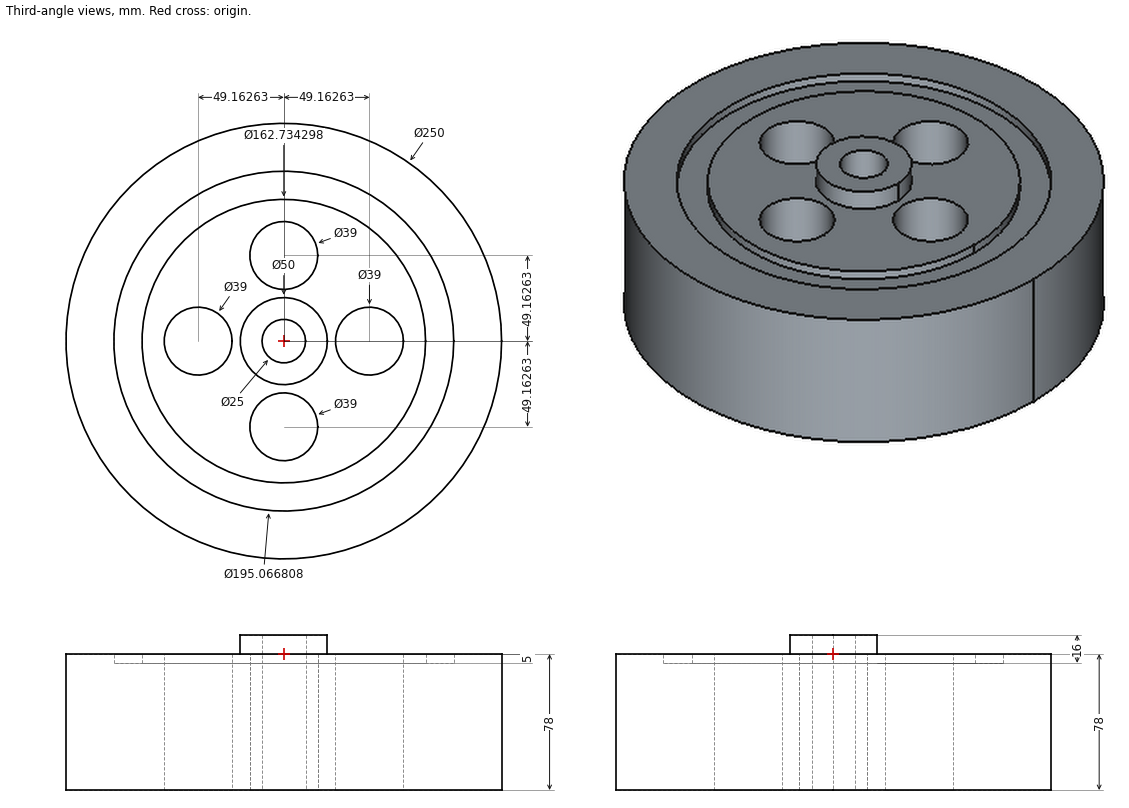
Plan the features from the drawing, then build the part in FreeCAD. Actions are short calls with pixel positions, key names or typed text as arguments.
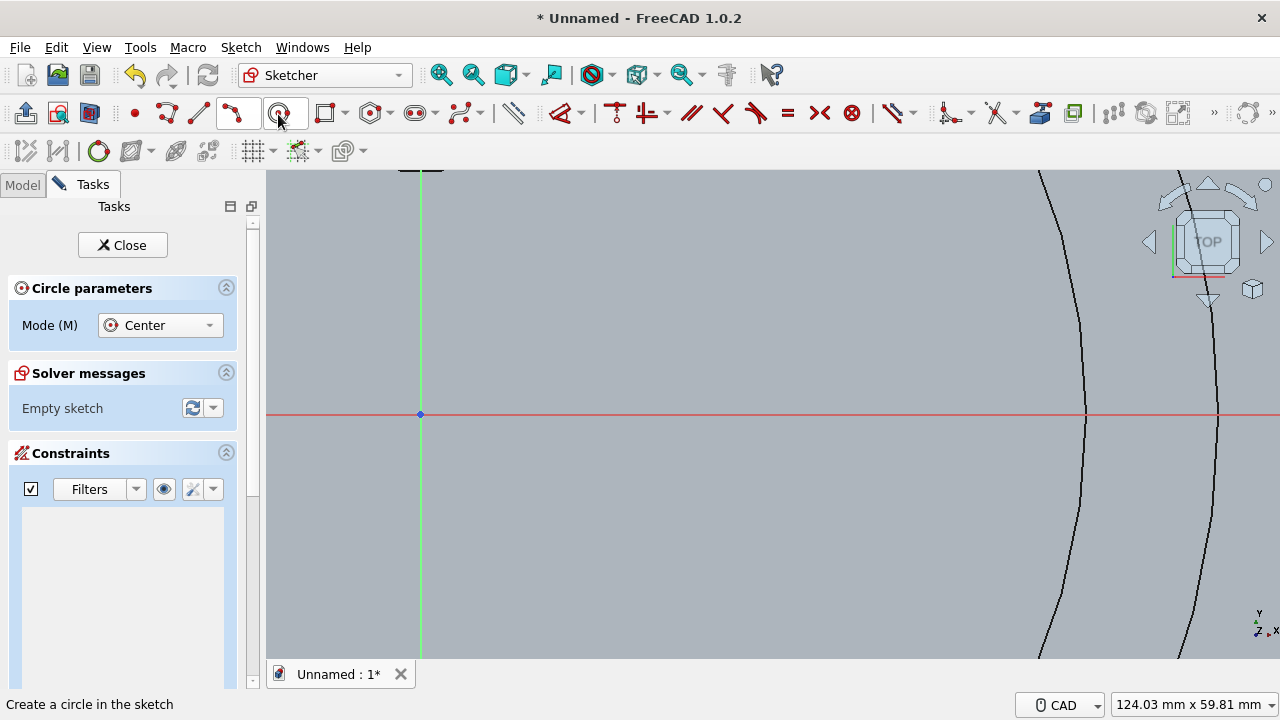
click(823, 414)
move(936, 302)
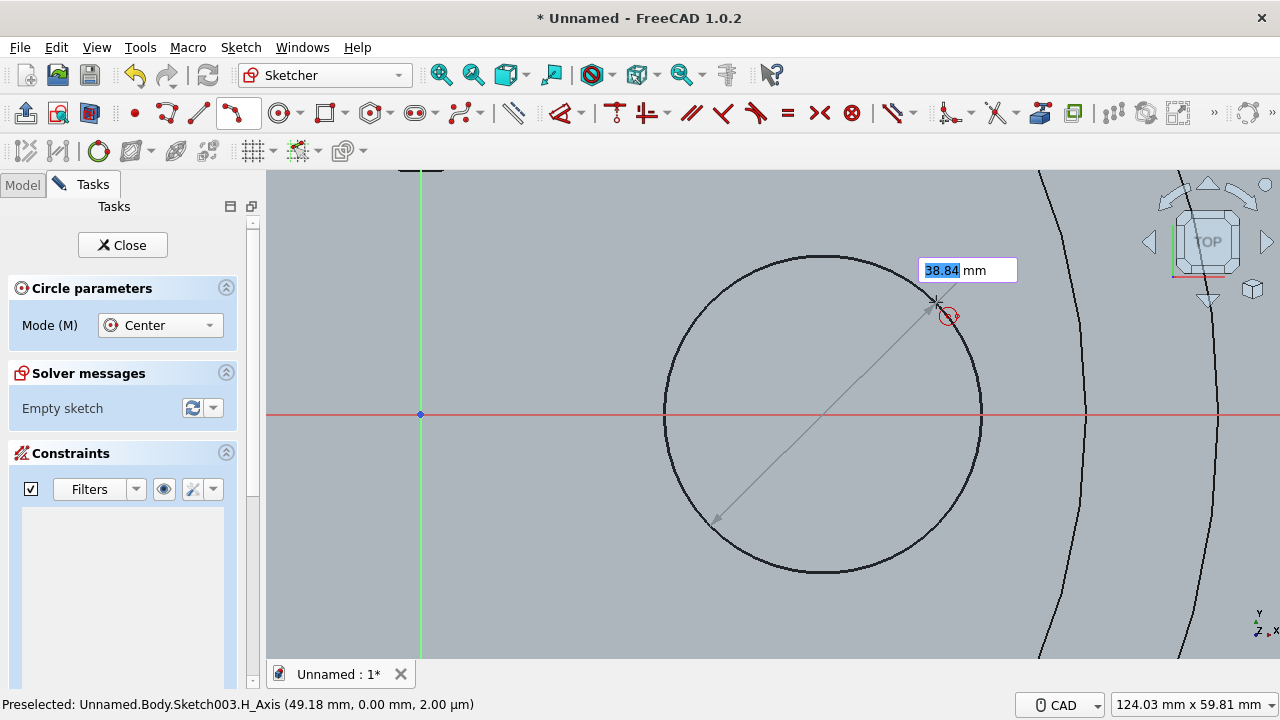
text(39)
key(Return)
key(Escape)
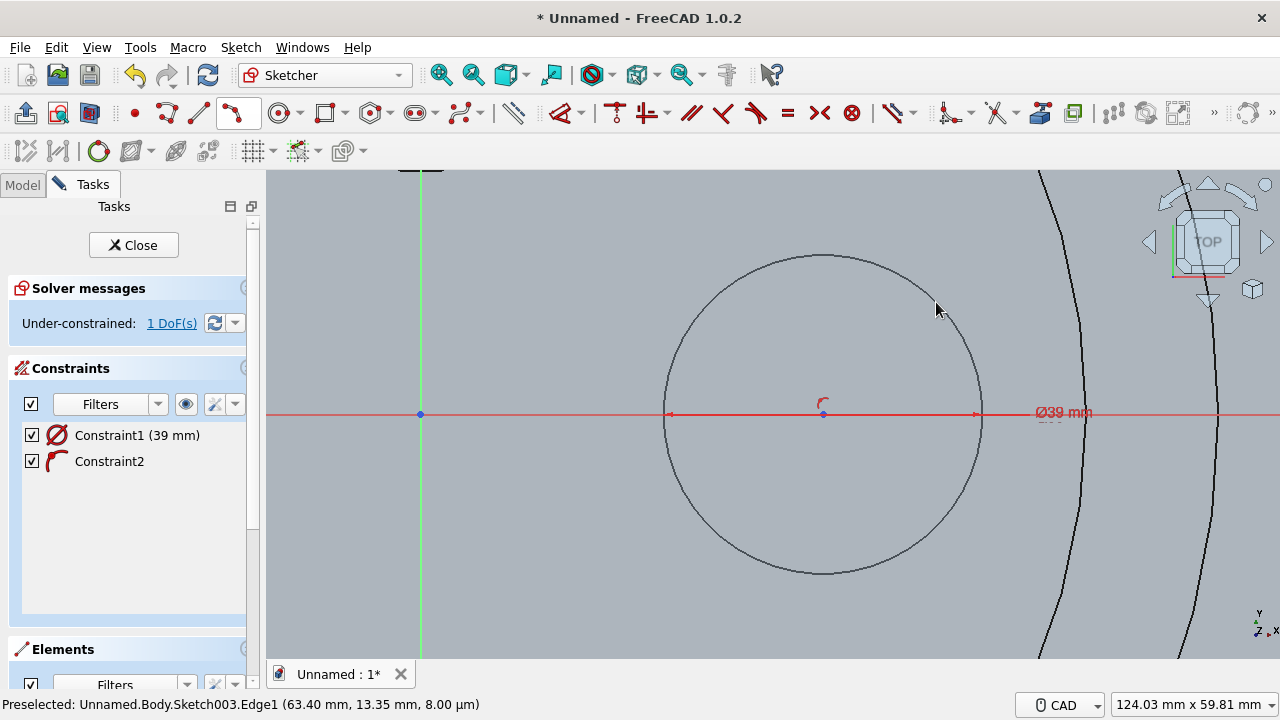
click(560, 114)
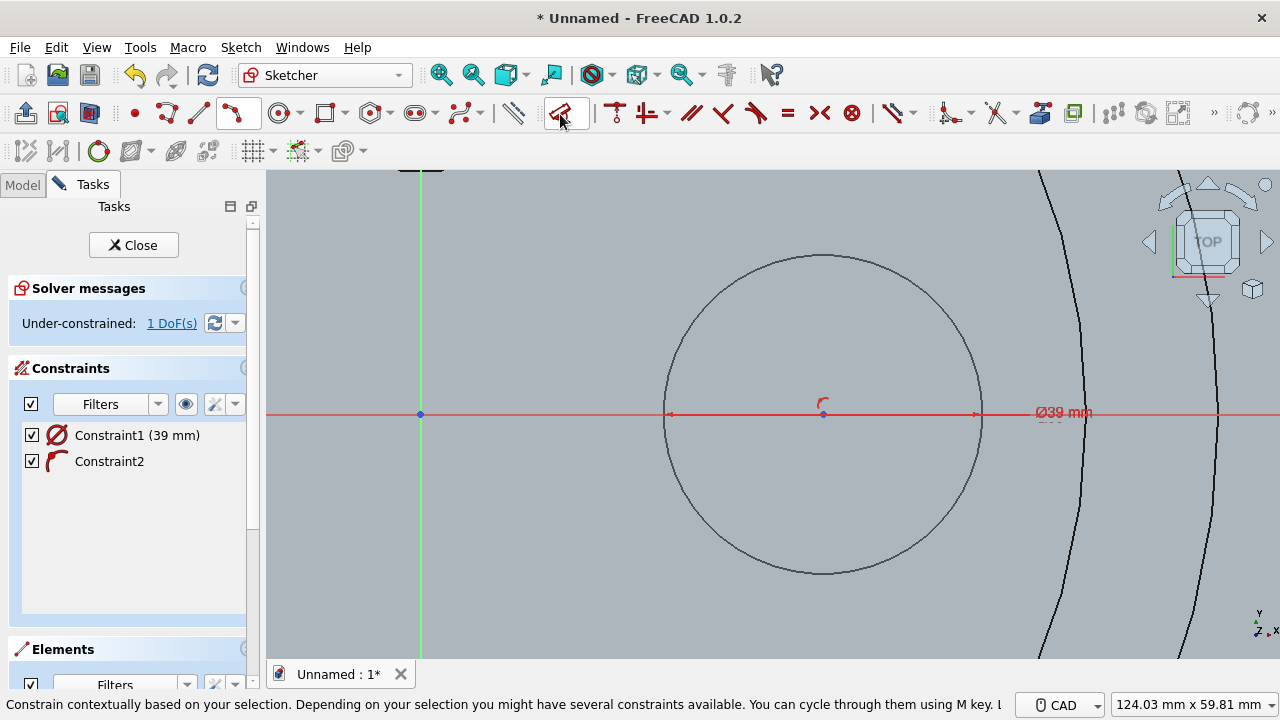
click(823, 414)
click(622, 448)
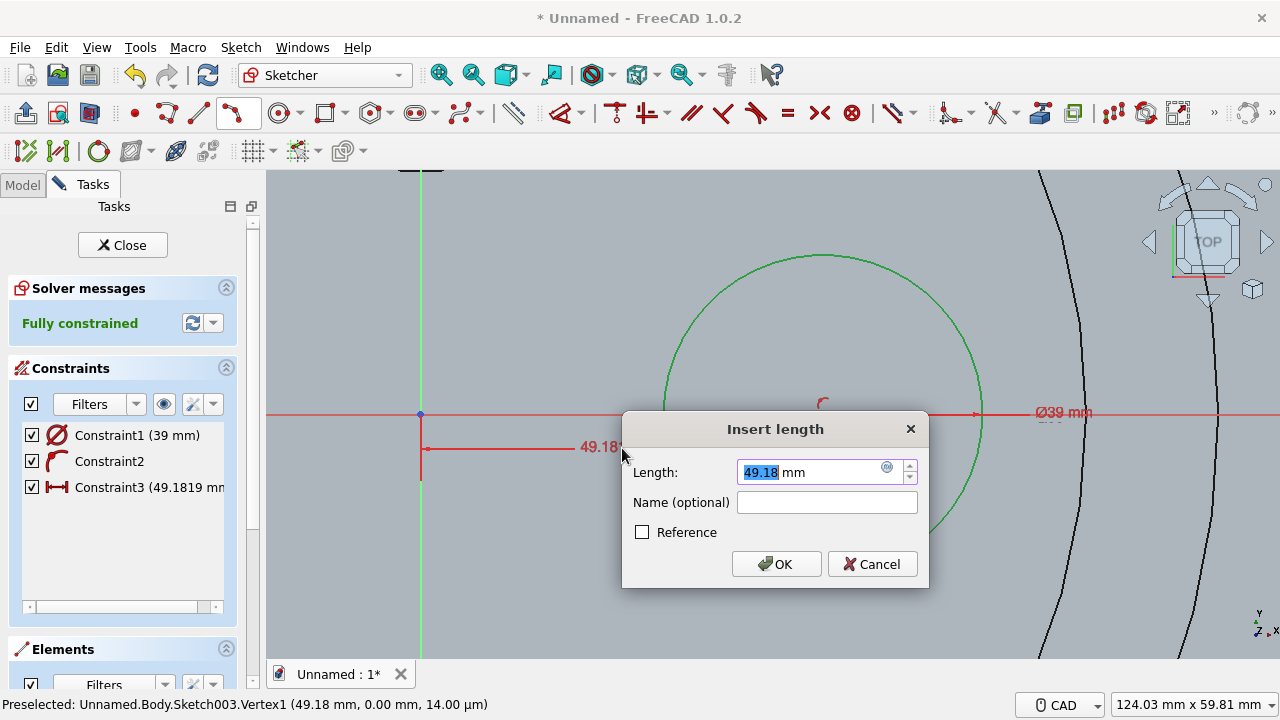
text(49.16263)
key(Return)
key(Escape)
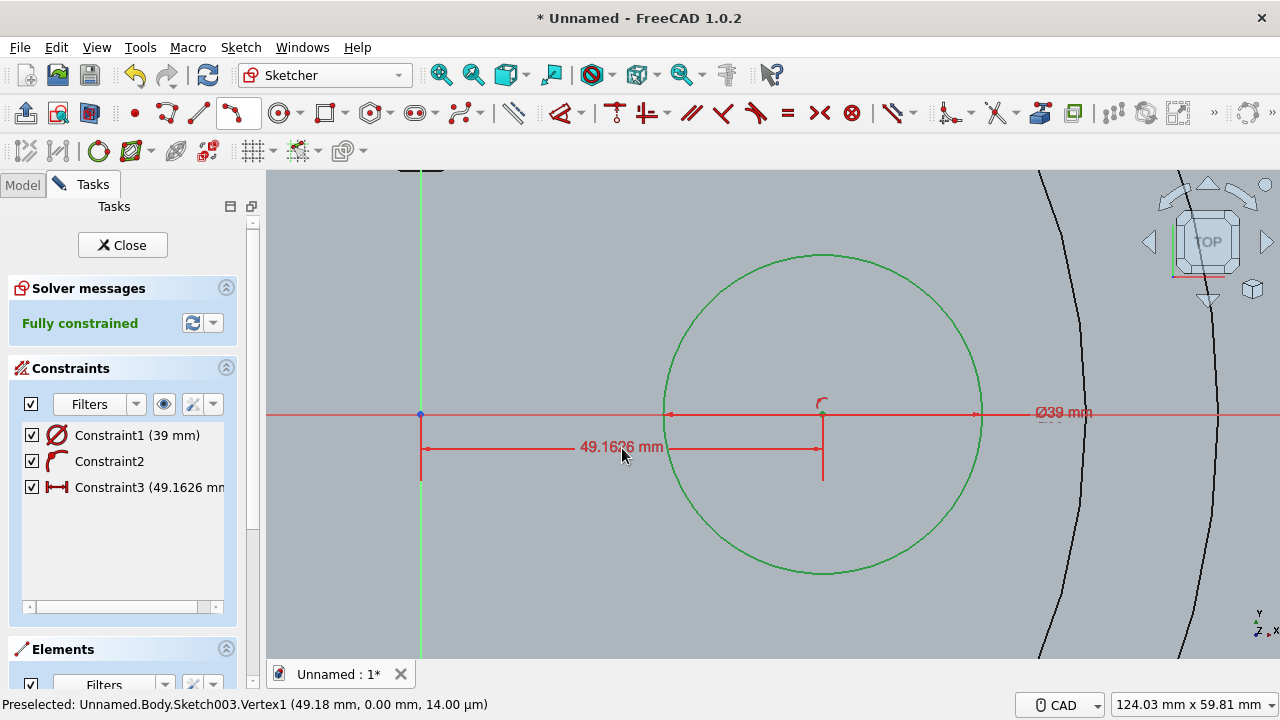
click(123, 245)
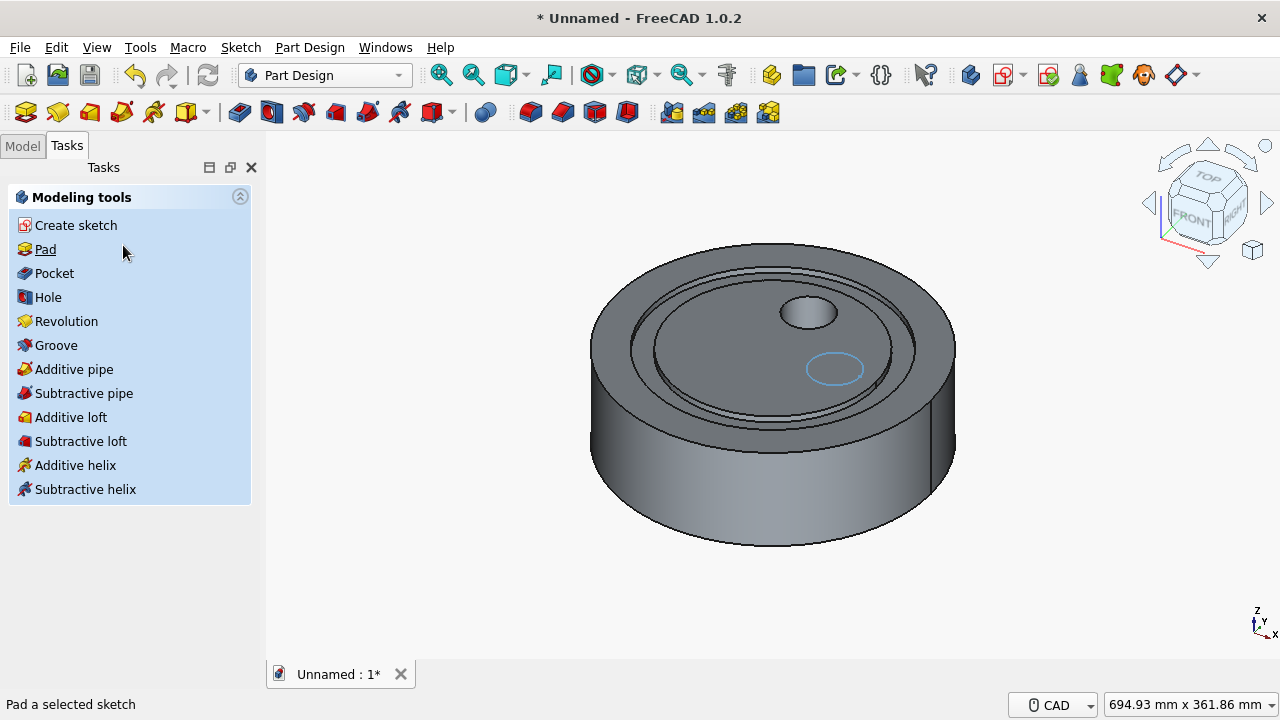
click(240, 112)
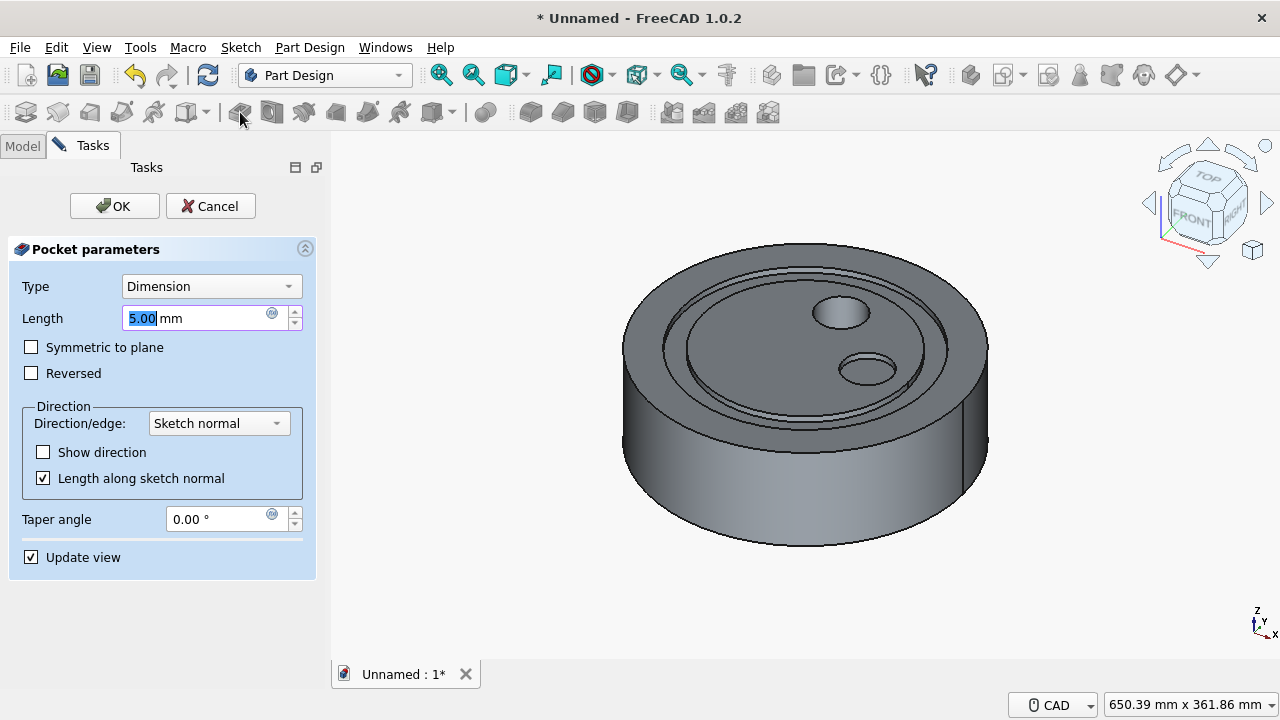
text(78)
key(Tab)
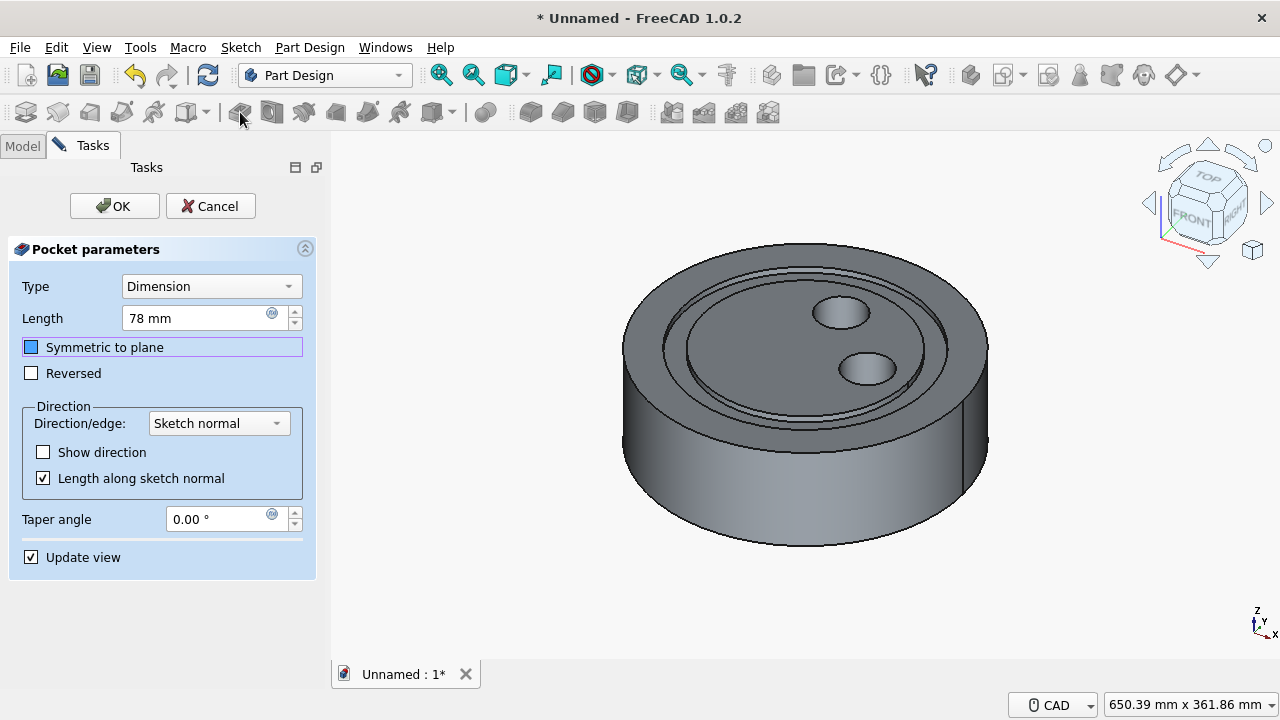
click(115, 206)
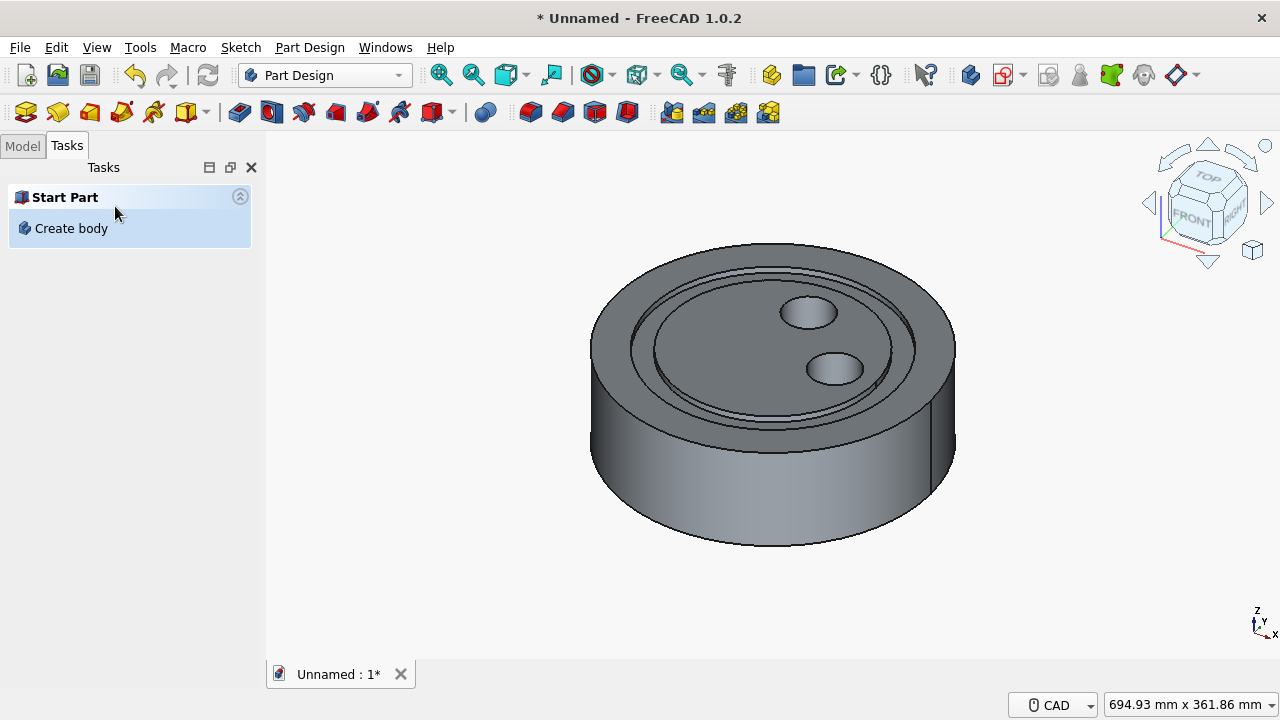
click(1004, 76)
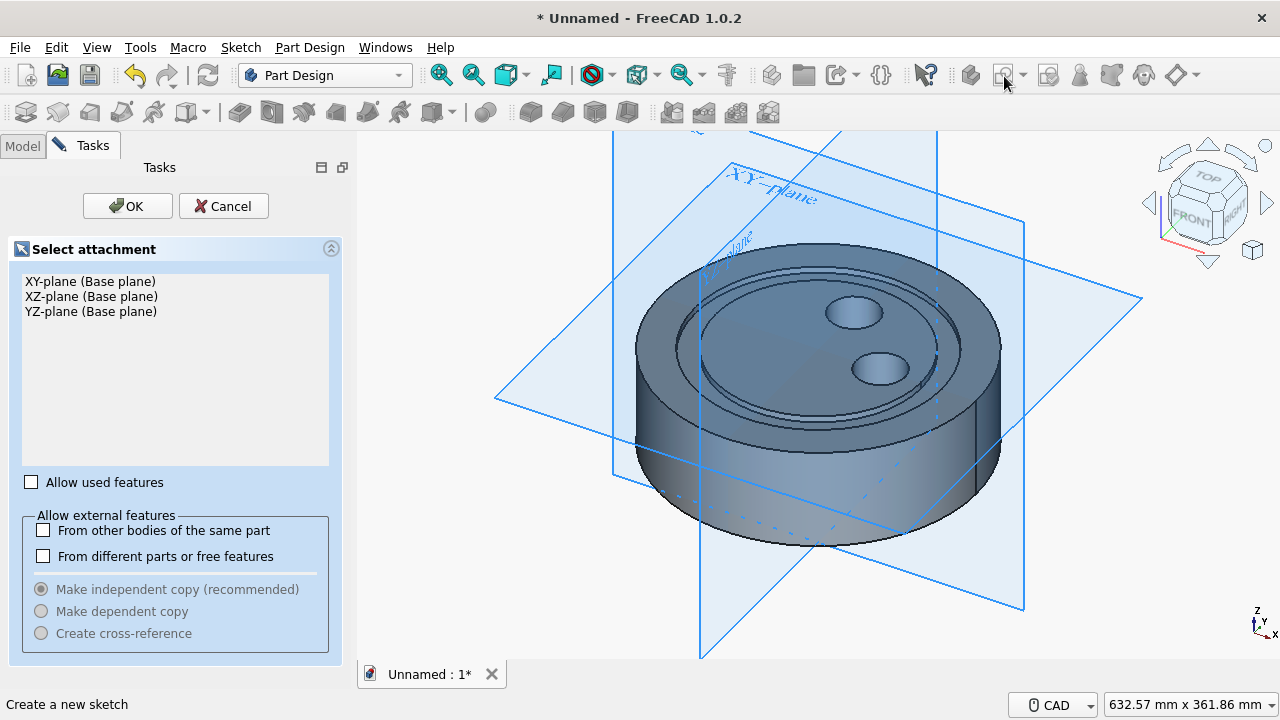
click(82, 282)